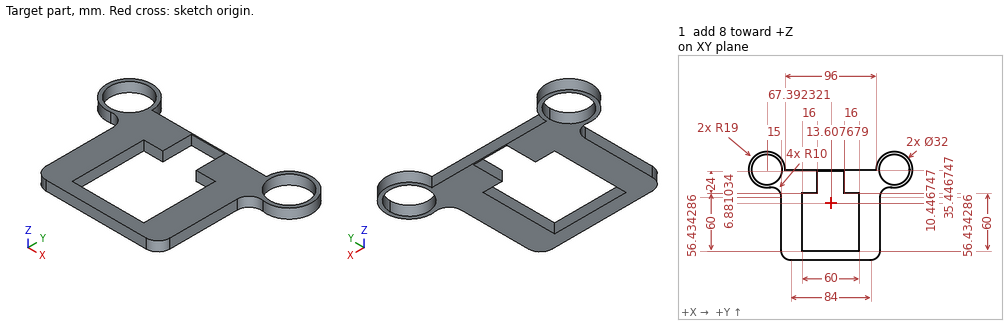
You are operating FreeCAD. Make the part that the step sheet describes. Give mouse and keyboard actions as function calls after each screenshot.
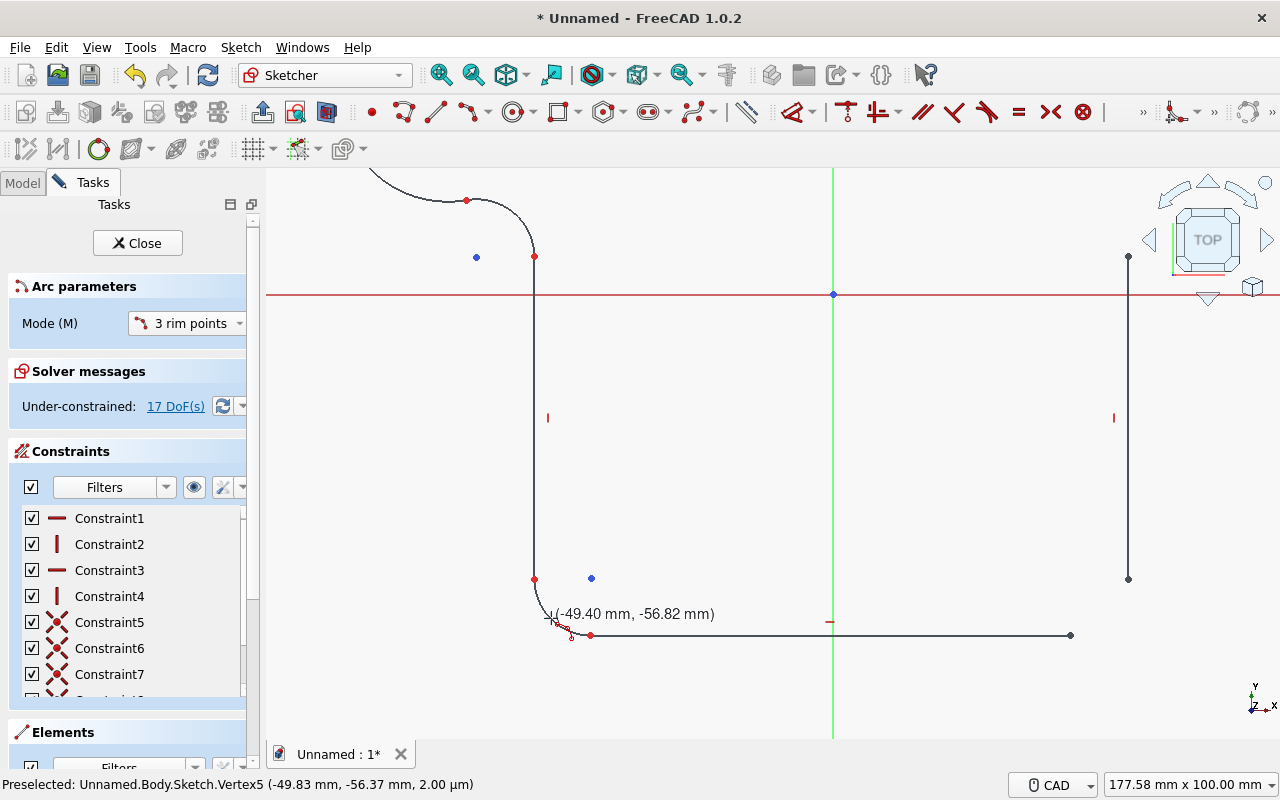
click(1070, 636)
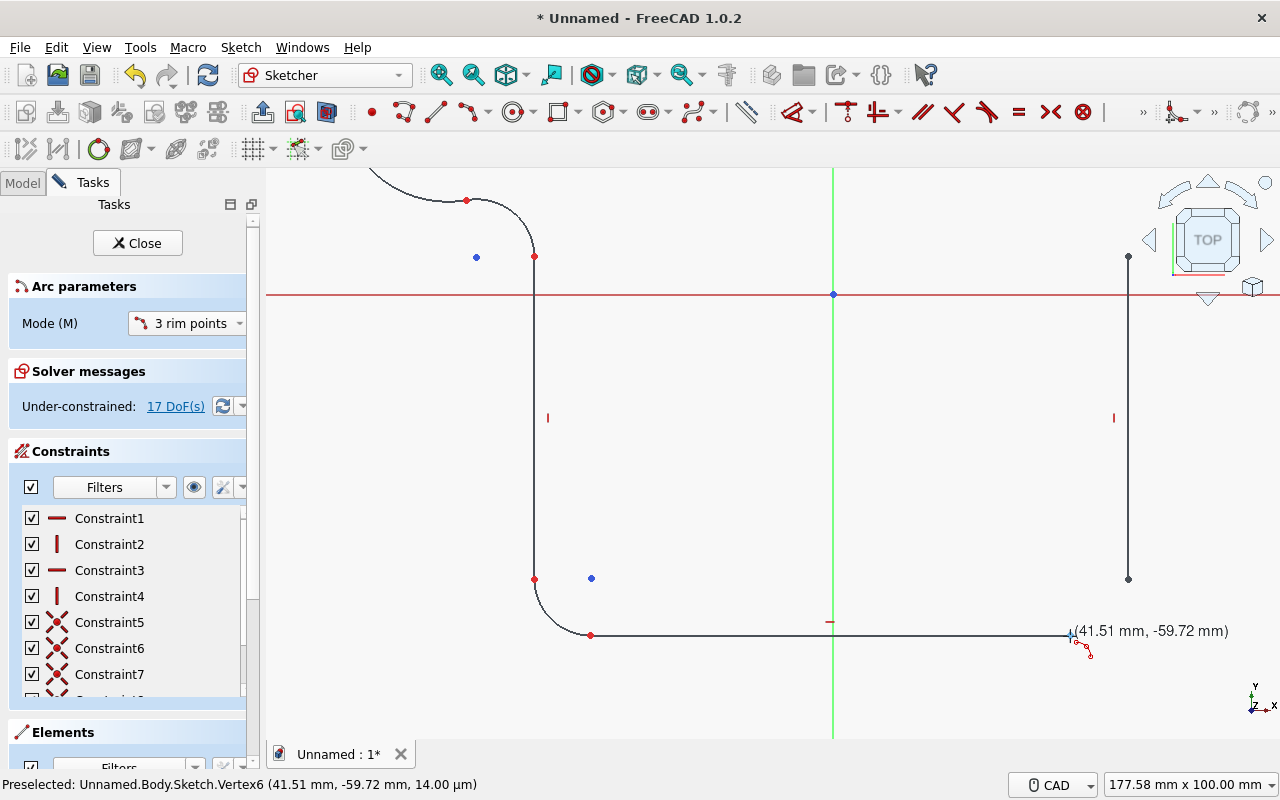
scroll(551, 619, down, 3)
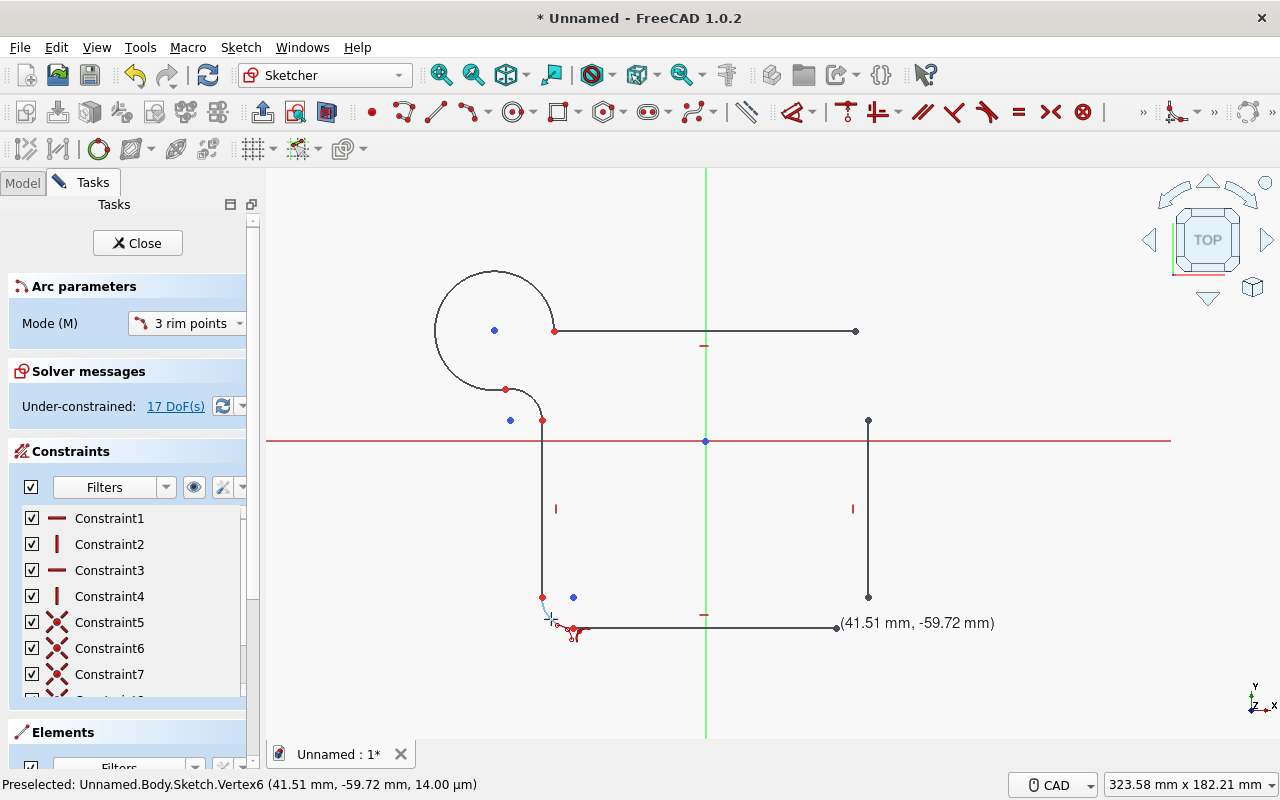
click(868, 597)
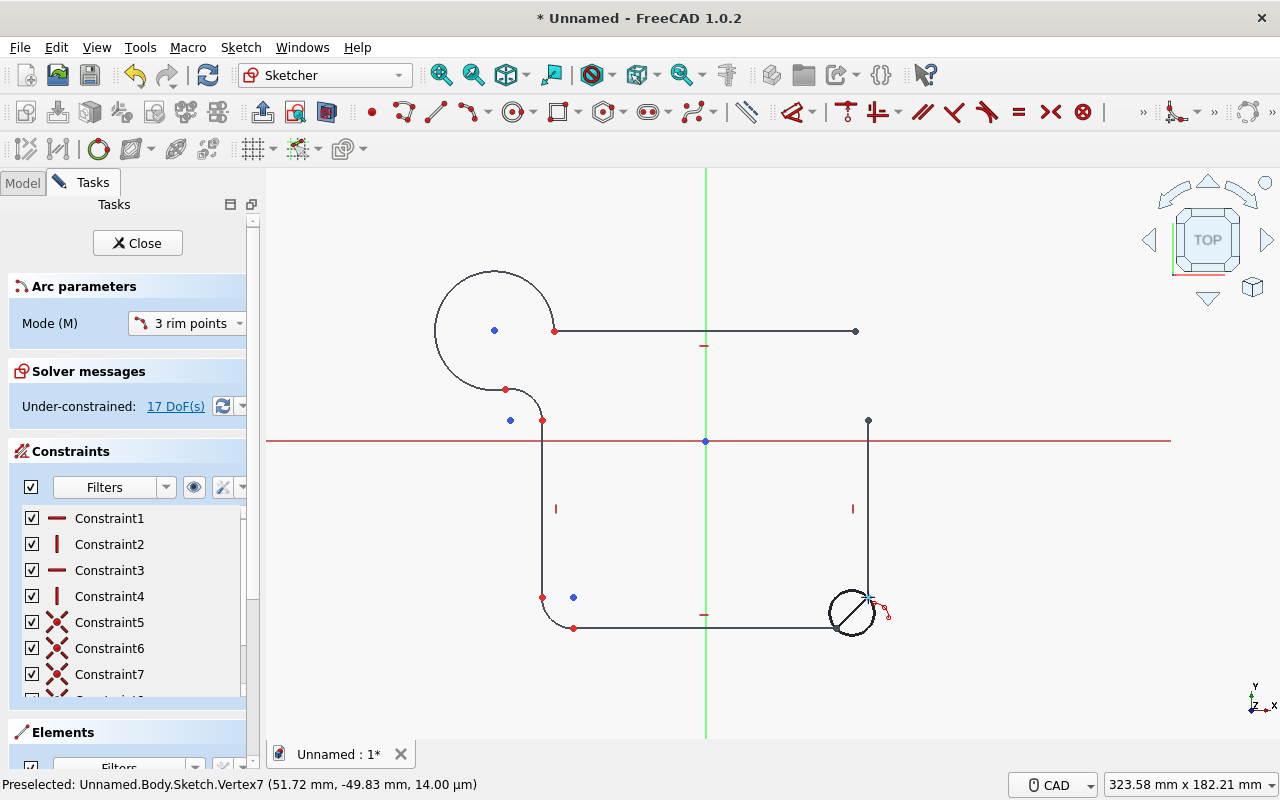
scroll(858, 619, up, 3)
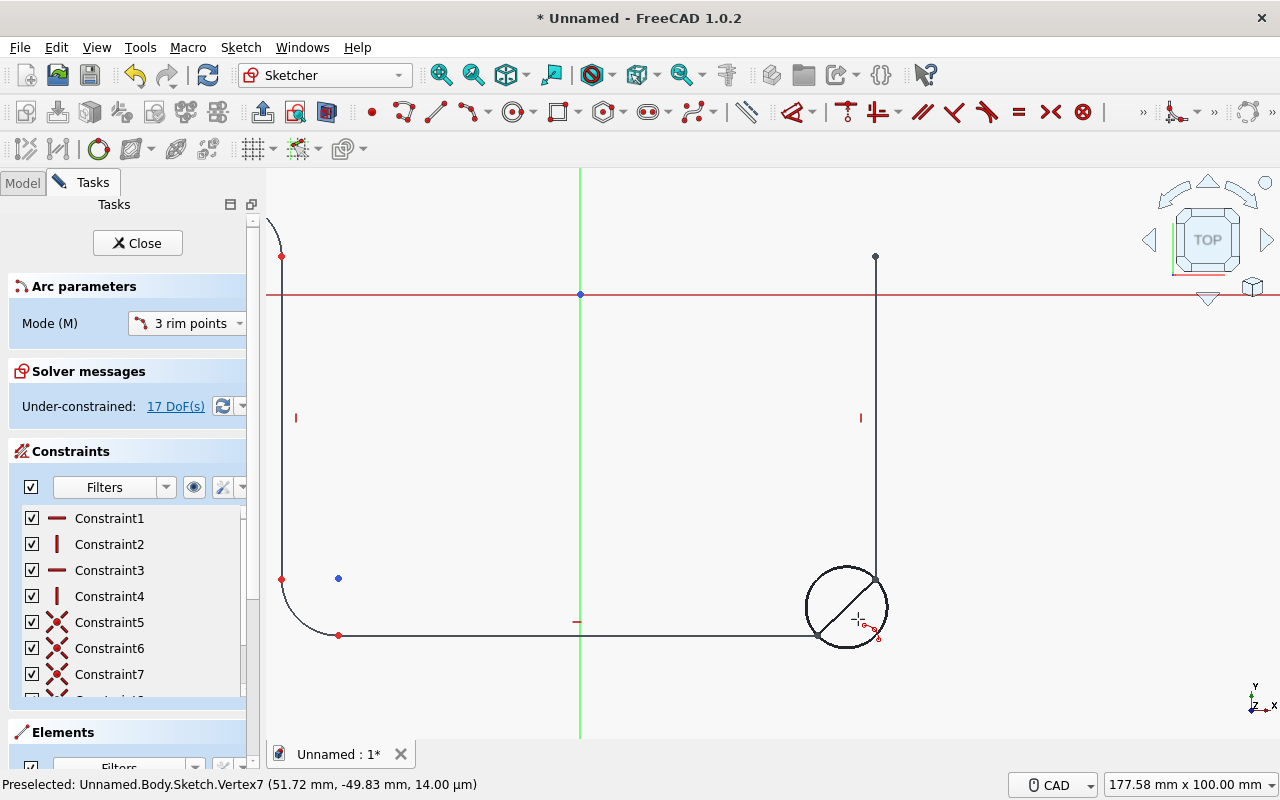
click(858, 618)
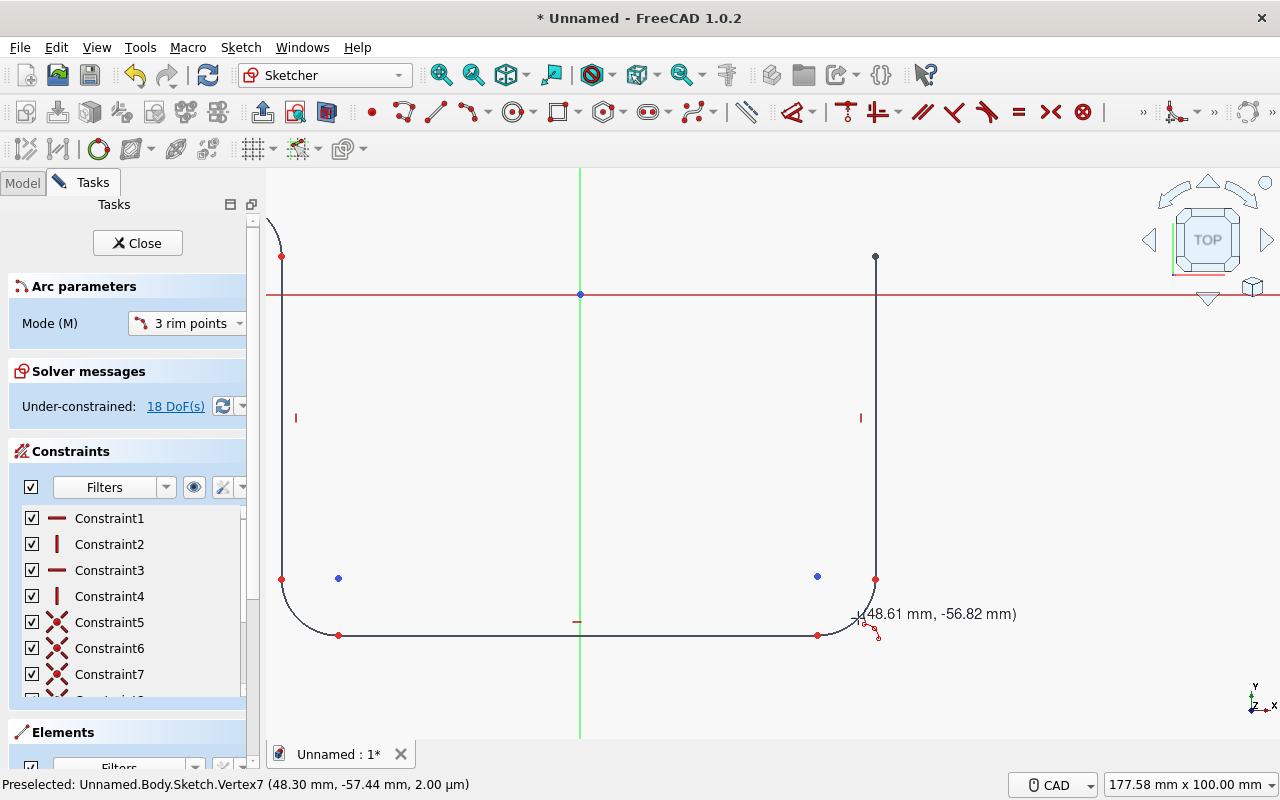
click(876, 257)
click(942, 199)
click(895, 212)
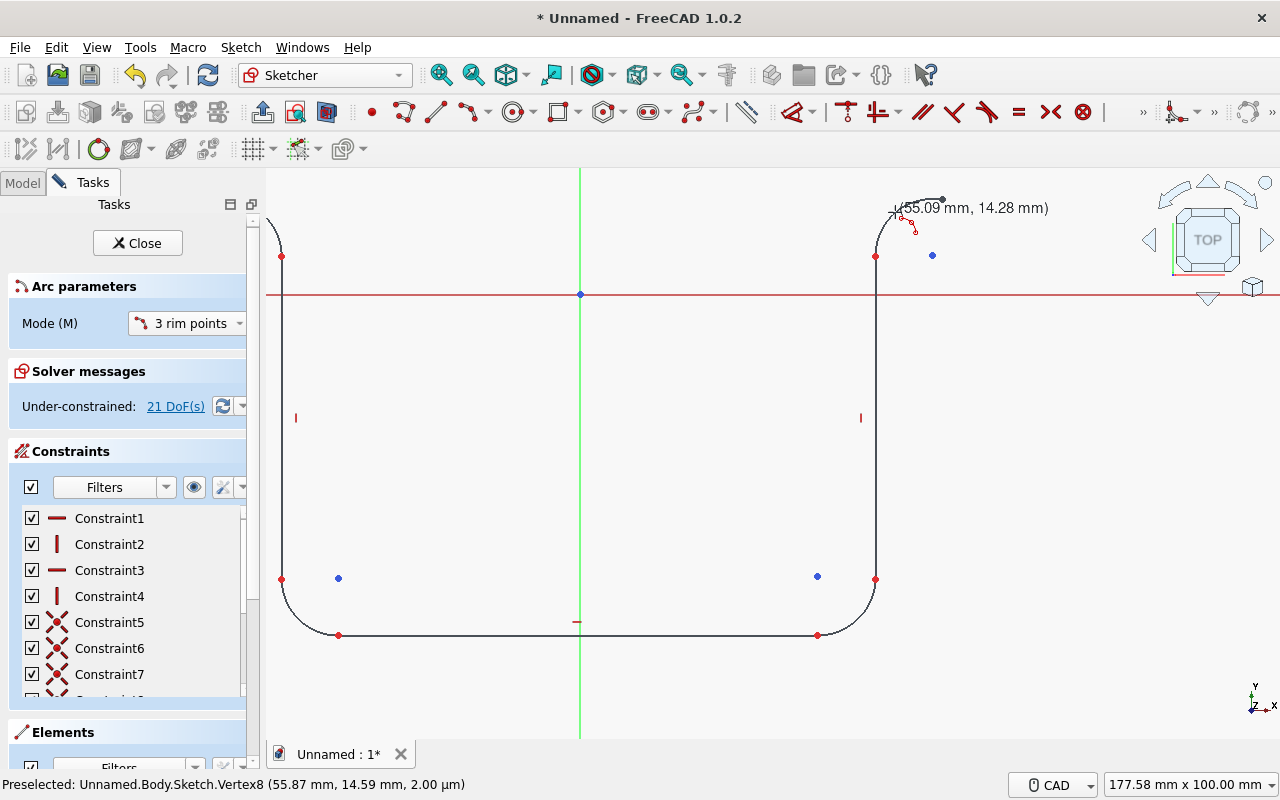
click(942, 200)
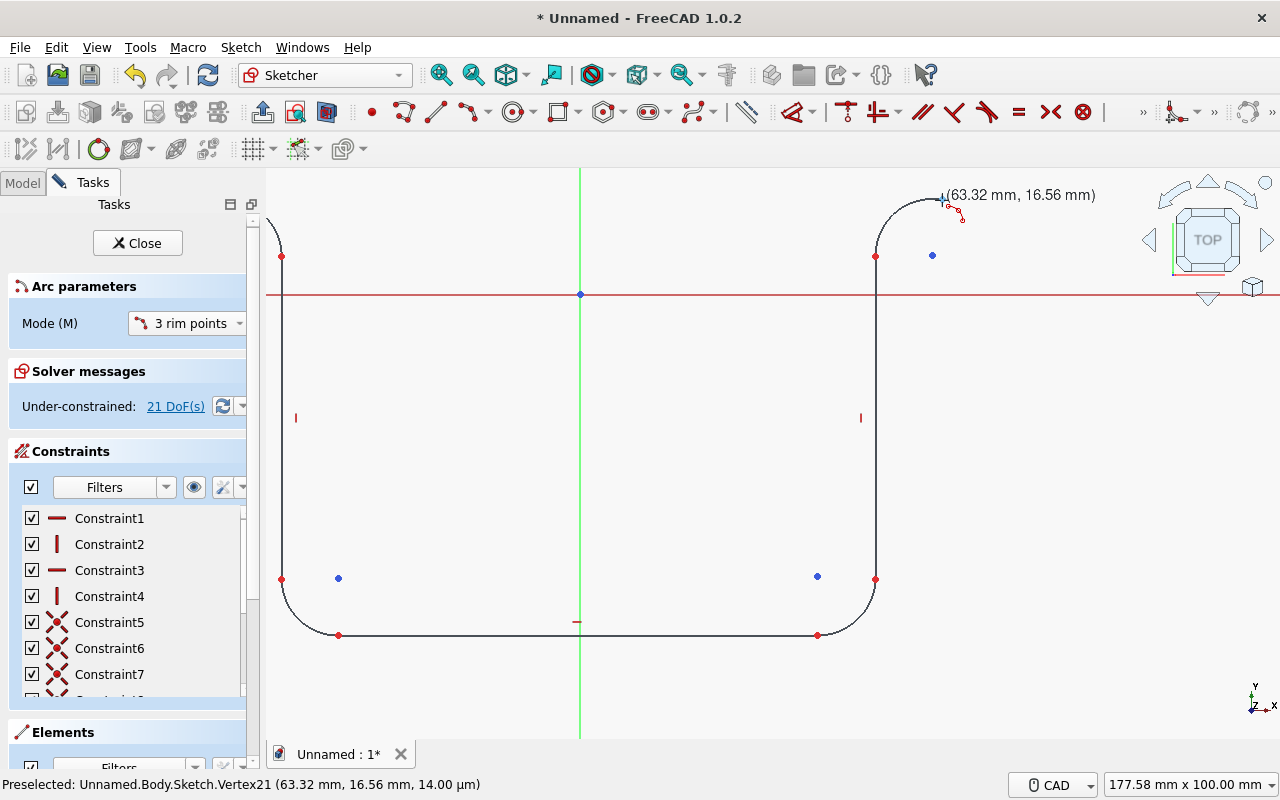
scroll(858, 619, down, 3)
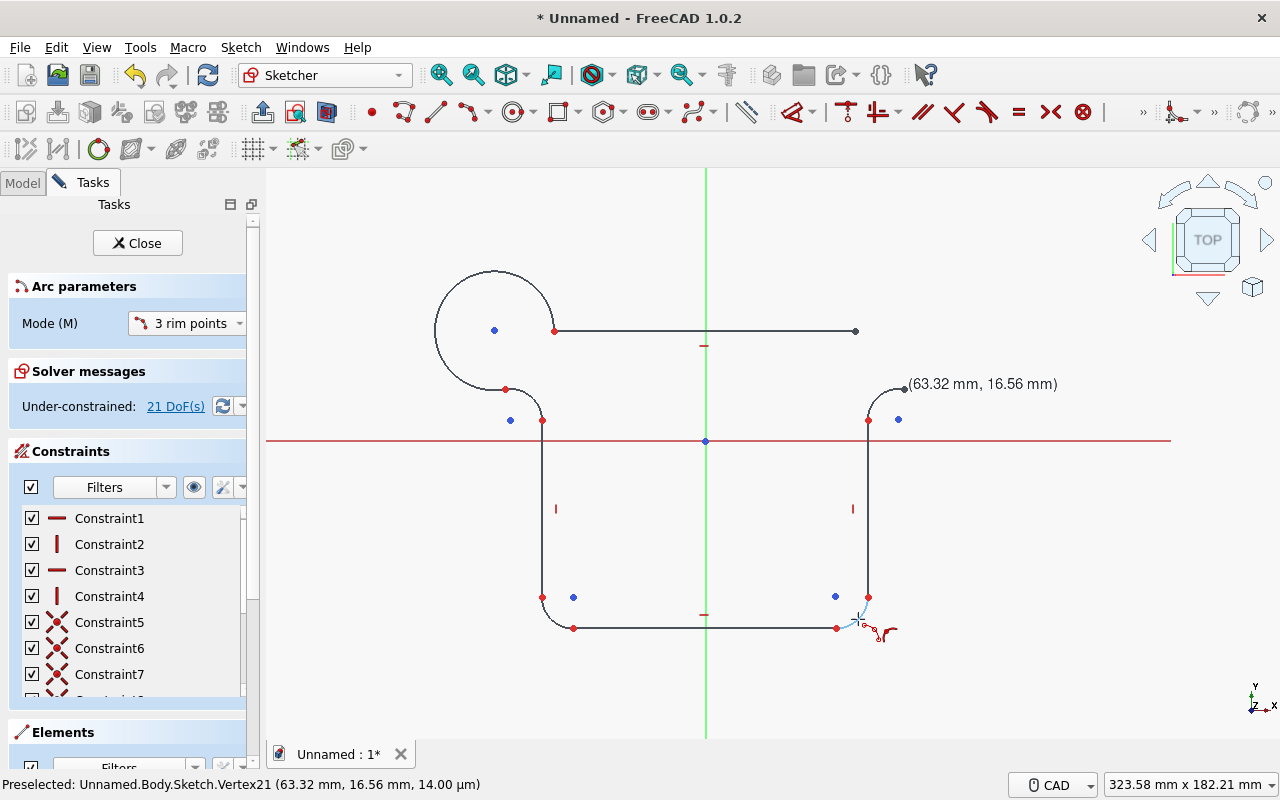
click(855, 331)
click(960, 292)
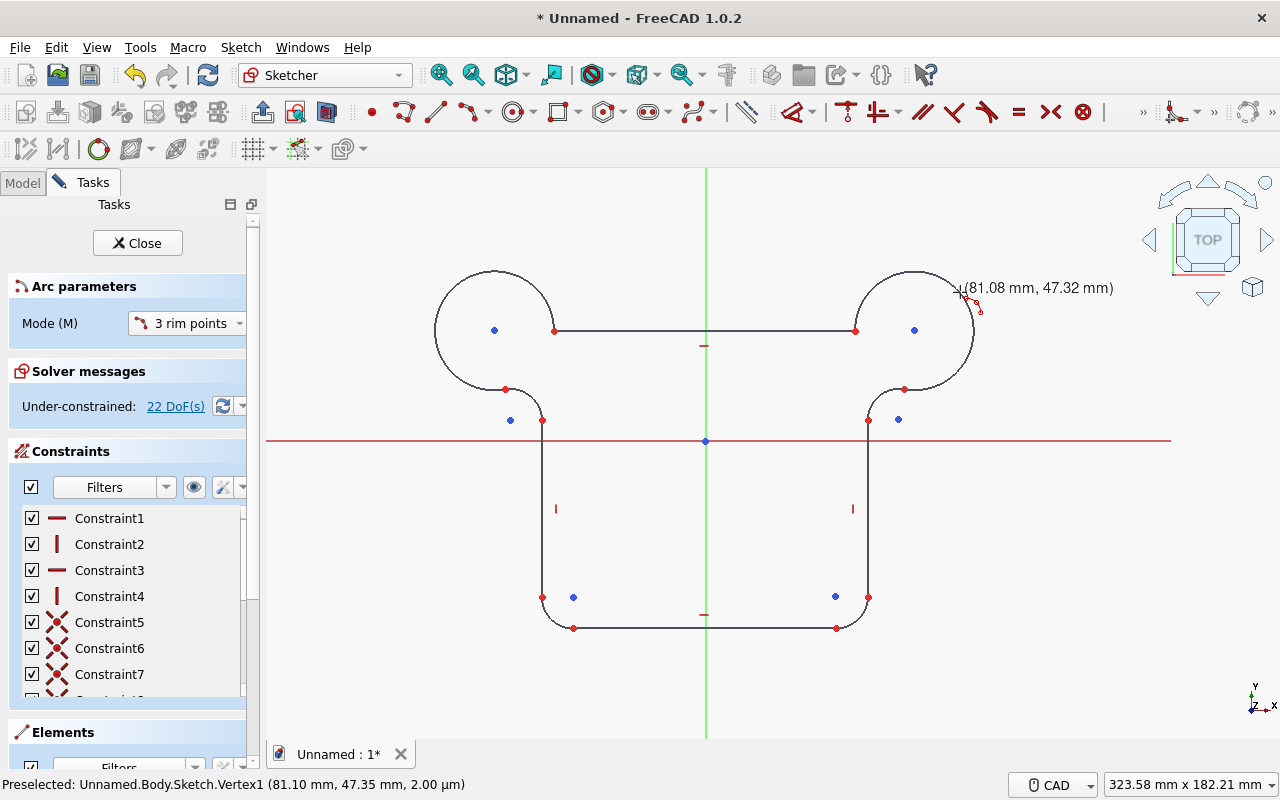
click(404, 112)